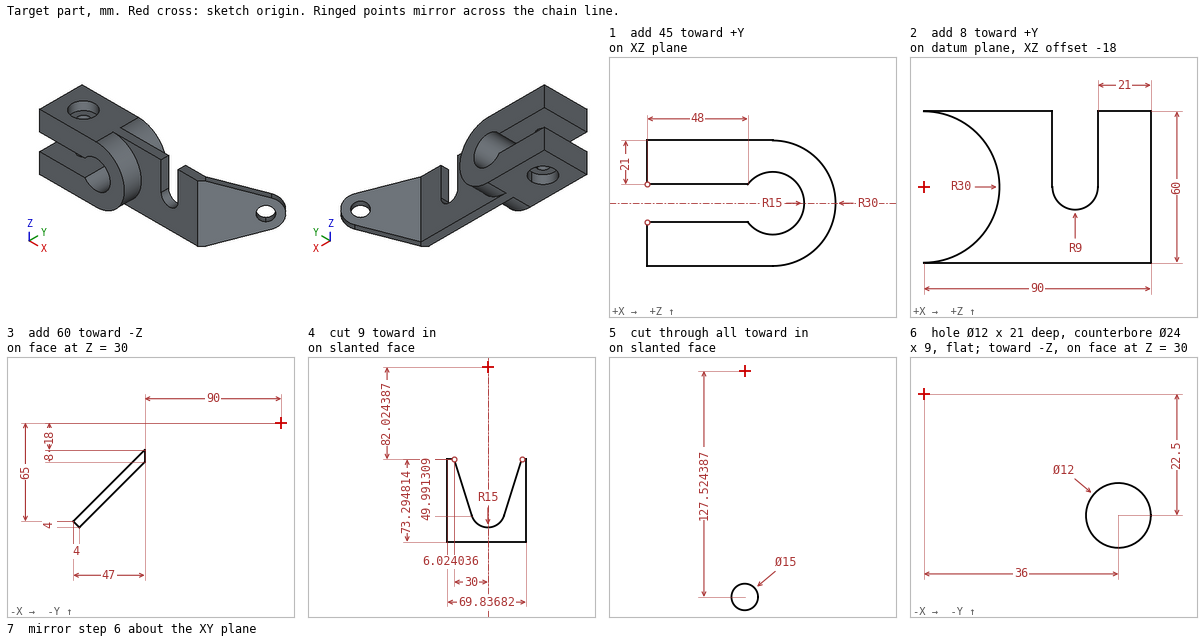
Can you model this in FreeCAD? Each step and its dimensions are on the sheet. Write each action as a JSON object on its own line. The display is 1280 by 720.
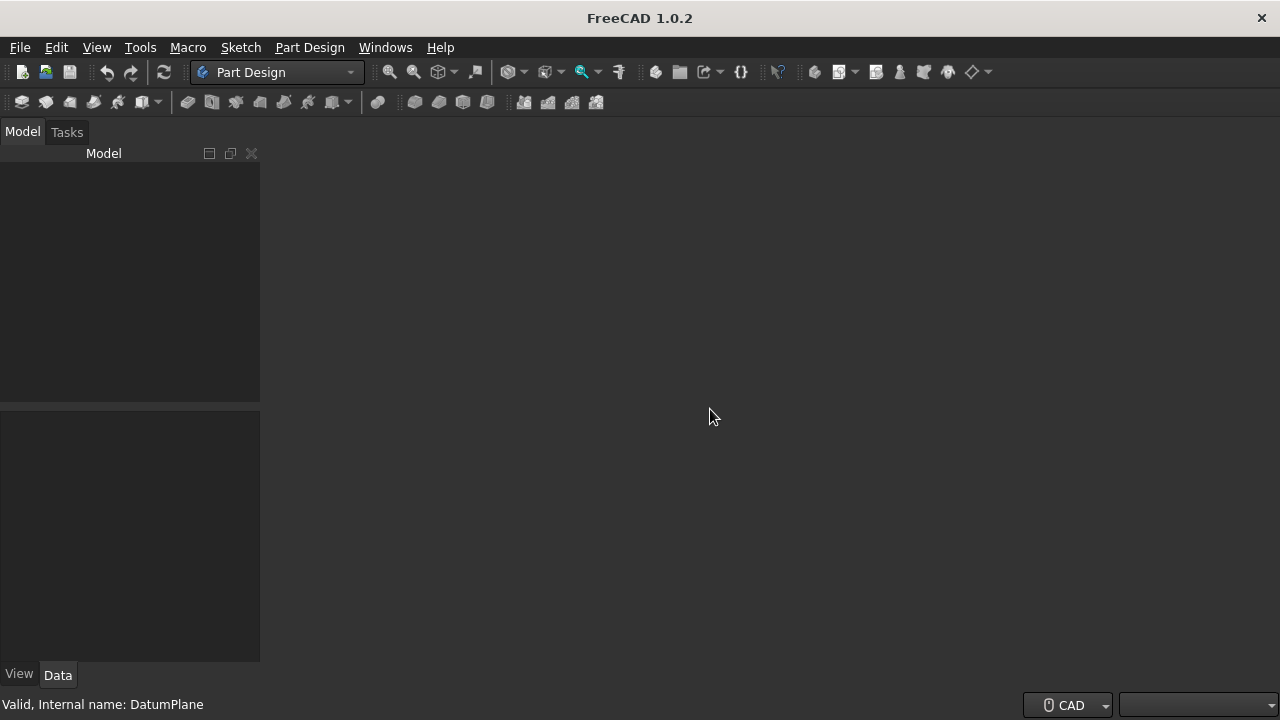
{"action": "left_click", "coordinate": [22, 72]}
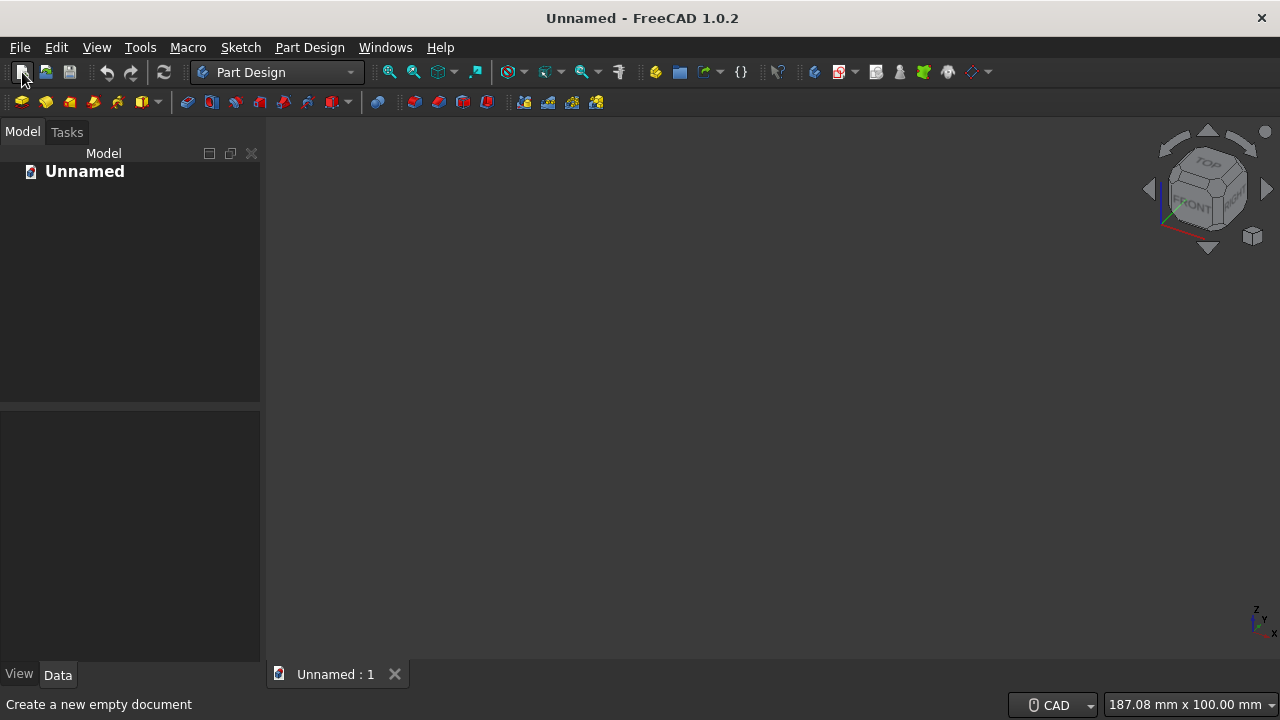
{"action": "left_click", "coordinate": [840, 72]}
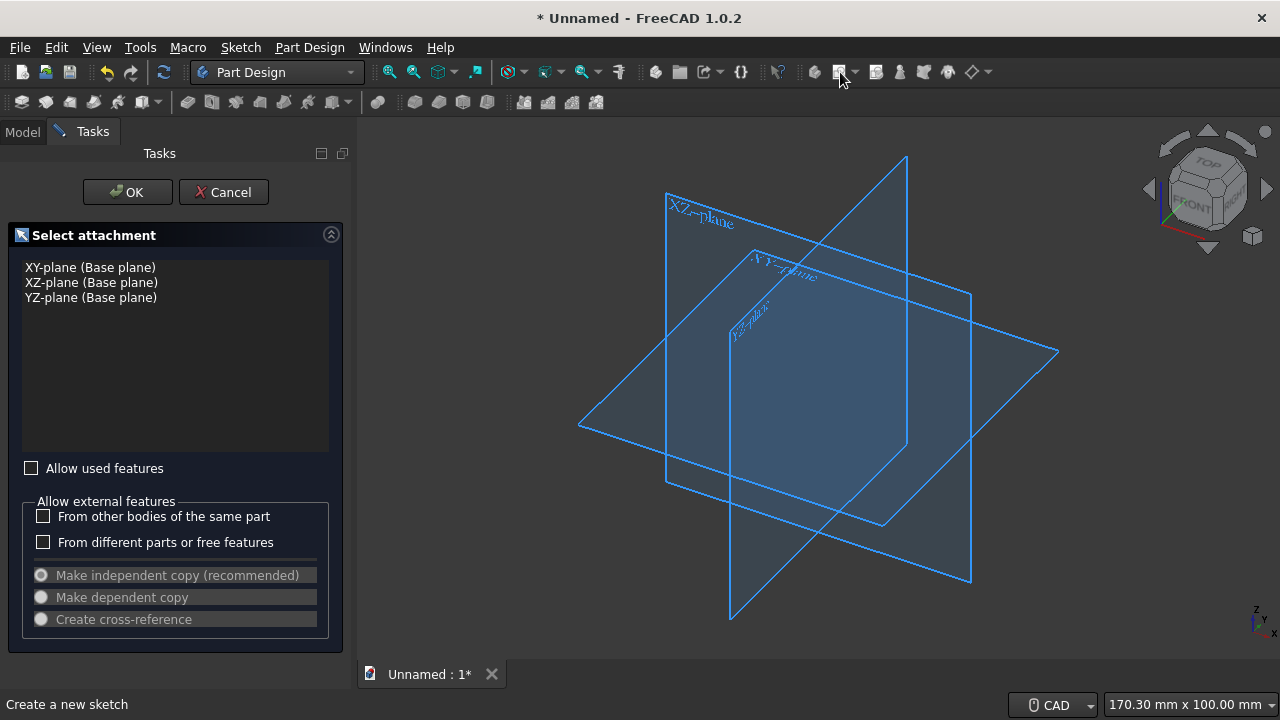
{"action": "left_click", "coordinate": [82, 282]}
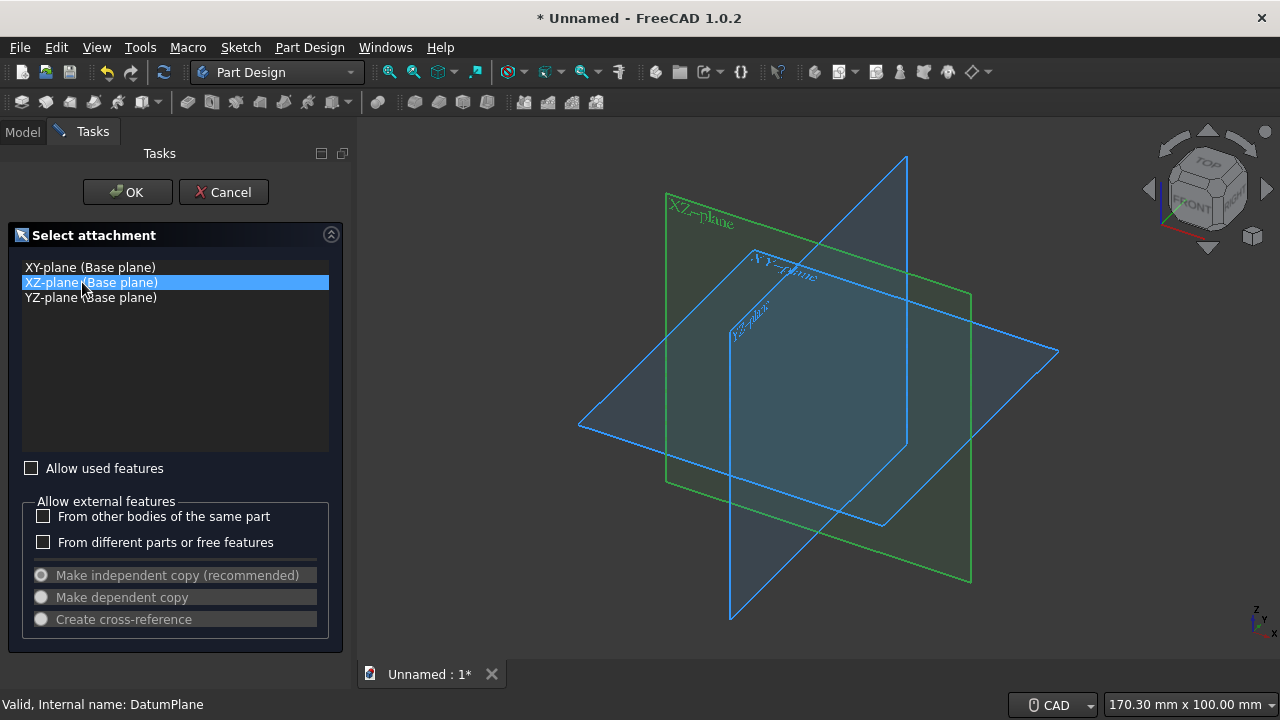
{"action": "left_click", "coordinate": [128, 192]}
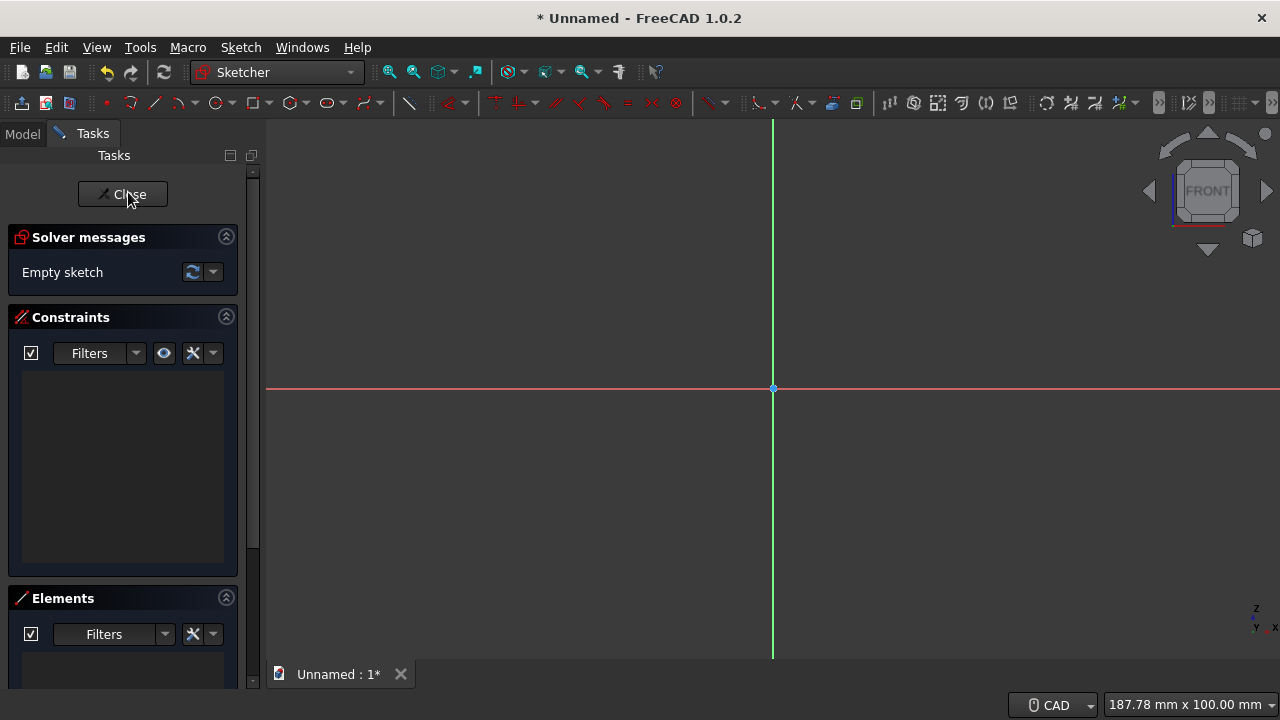
{"action": "left_click", "coordinate": [132, 104]}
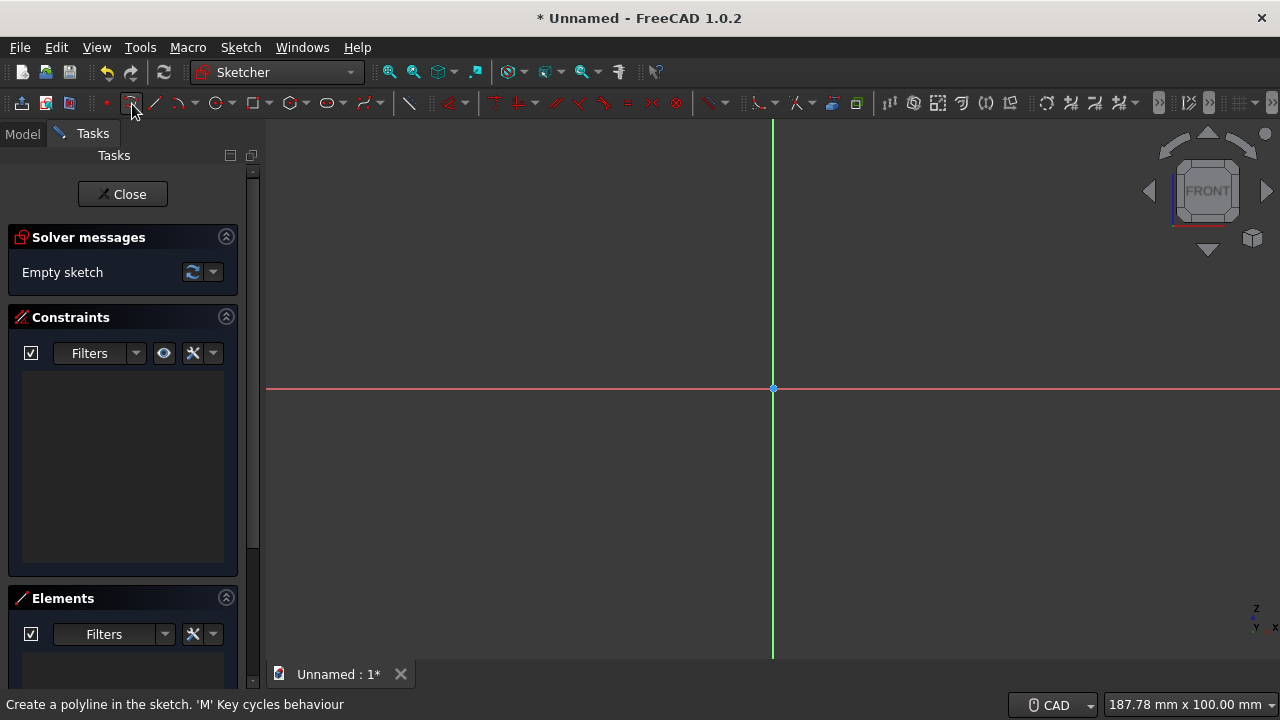
{"action": "left_click", "coordinate": [708, 340]}
{"action": "left_click", "coordinate": [449, 340]}
{"action": "left_click", "coordinate": [449, 227]}
{"action": "left_click", "coordinate": [773, 227]}
{"action": "right_click", "coordinate": [773, 227]}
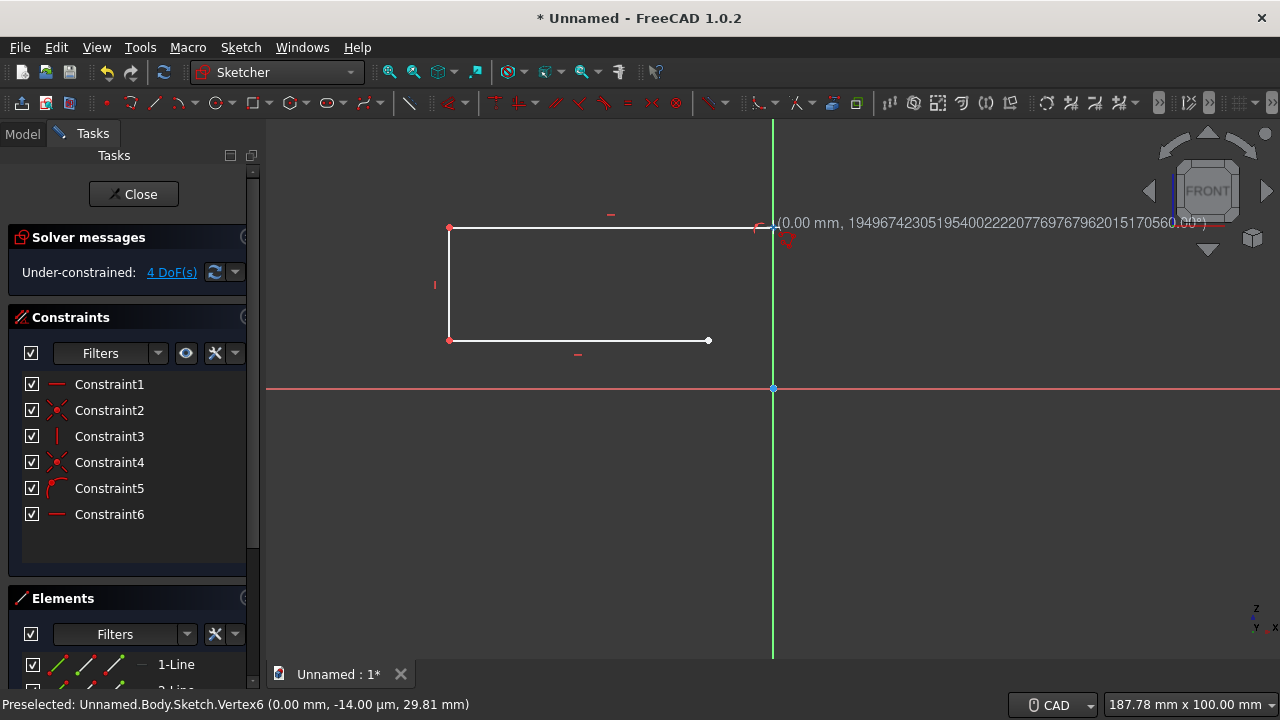
{"action": "left_click", "coordinate": [773, 551]}
{"action": "left_click", "coordinate": [449, 551]}
{"action": "left_click", "coordinate": [449, 438]}
{"action": "left_click", "coordinate": [708, 438]}
{"action": "right_click", "coordinate": [708, 438]}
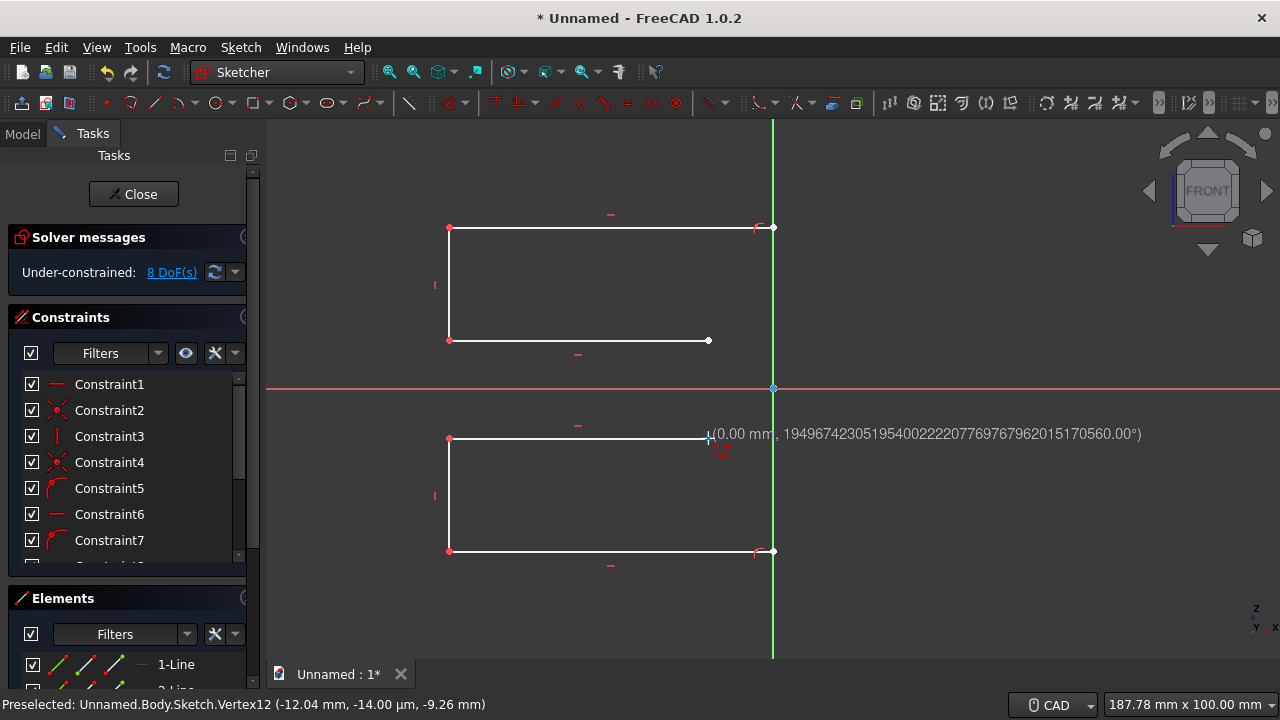
{"action": "left_click", "coordinate": [198, 104]}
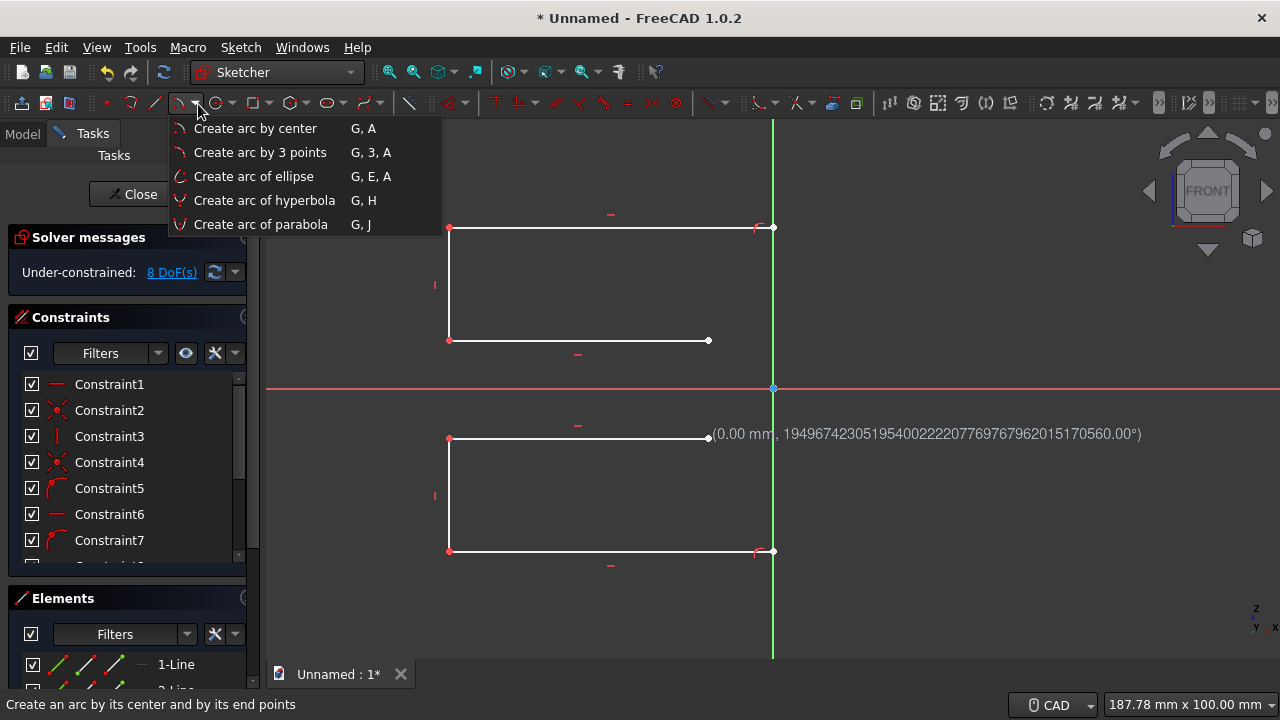
{"action": "left_click", "coordinate": [306, 152]}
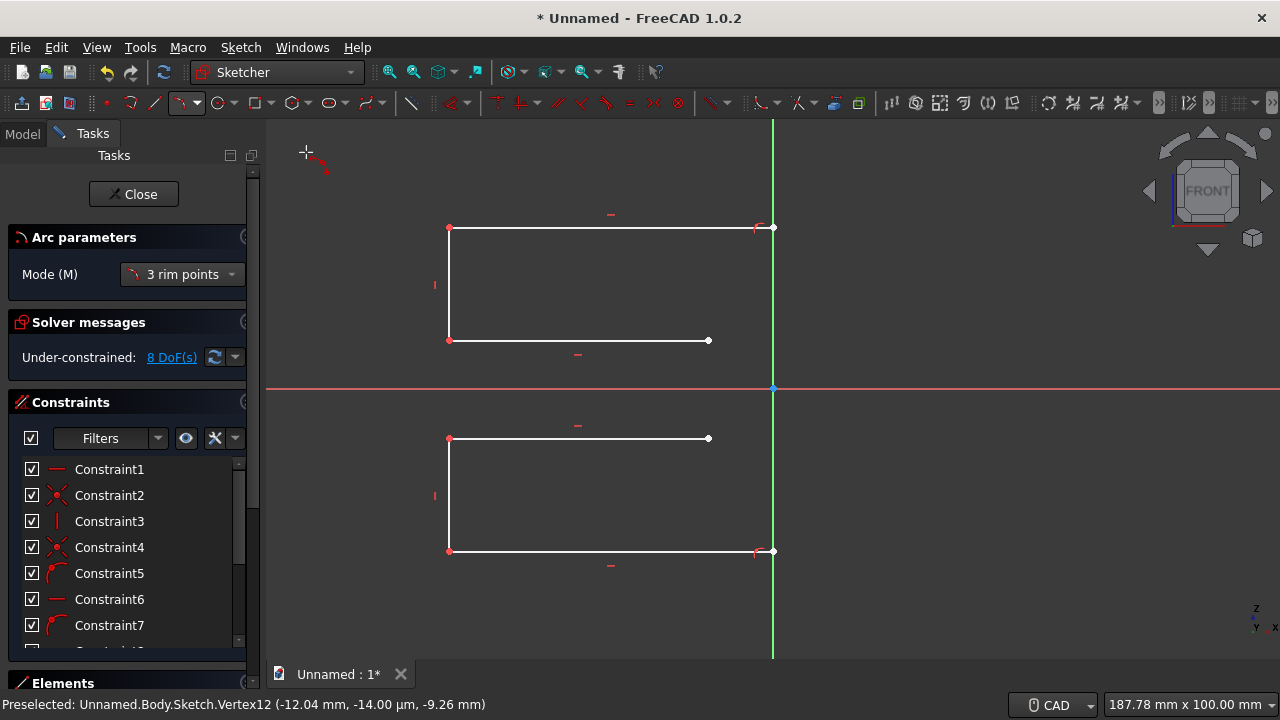
{"action": "left_click", "coordinate": [773, 228]}
{"action": "left_click", "coordinate": [773, 552]}
{"action": "left_click", "coordinate": [927, 439]}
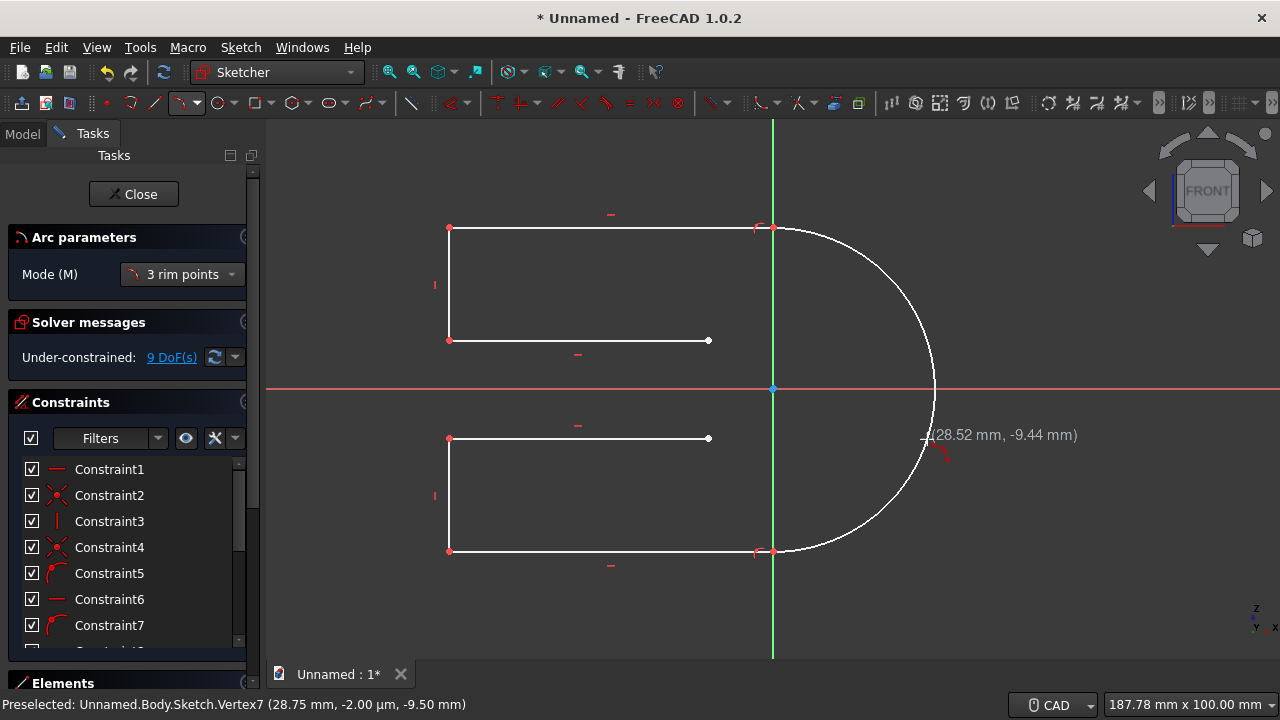
{"action": "left_click", "coordinate": [708, 439]}
{"action": "left_click", "coordinate": [708, 341]}
{"action": "left_click", "coordinate": [844, 428]}
{"action": "key", "text": "Escape"}